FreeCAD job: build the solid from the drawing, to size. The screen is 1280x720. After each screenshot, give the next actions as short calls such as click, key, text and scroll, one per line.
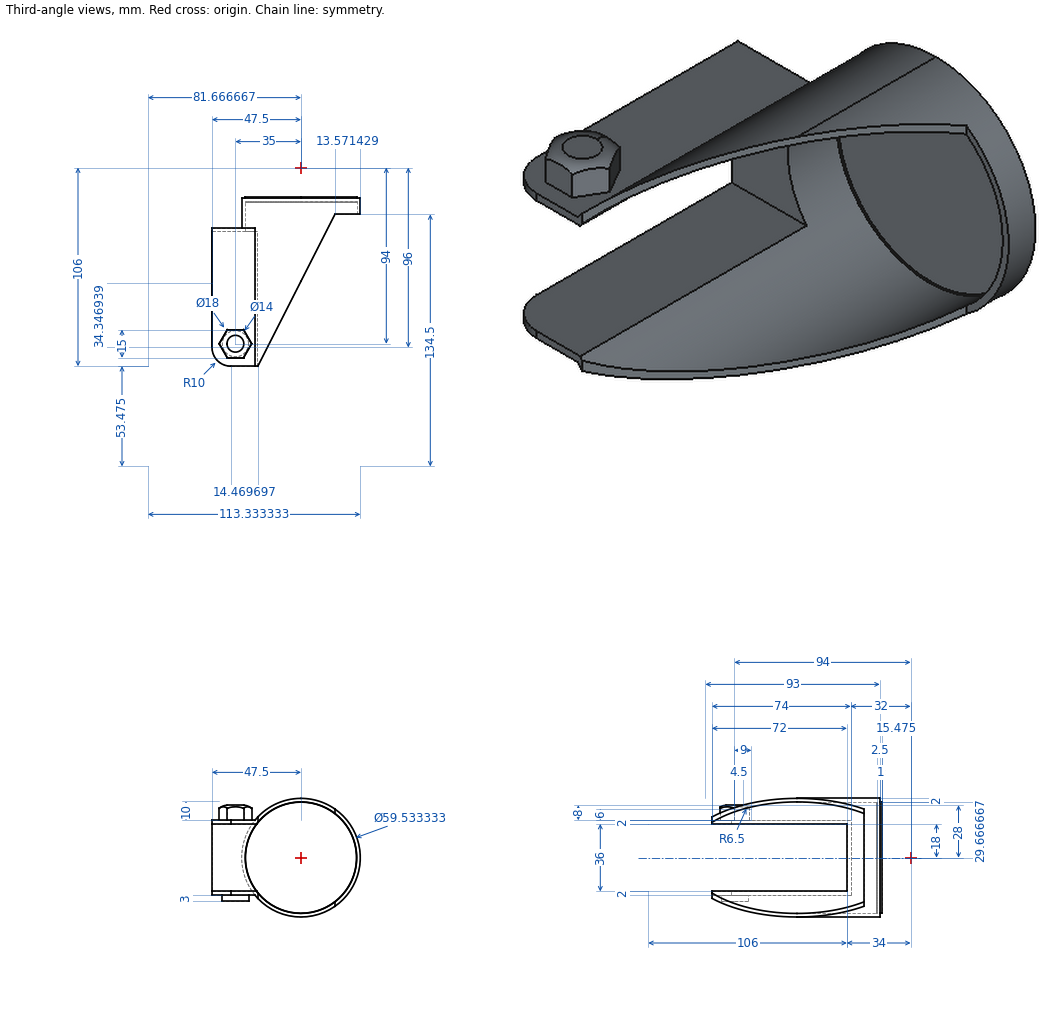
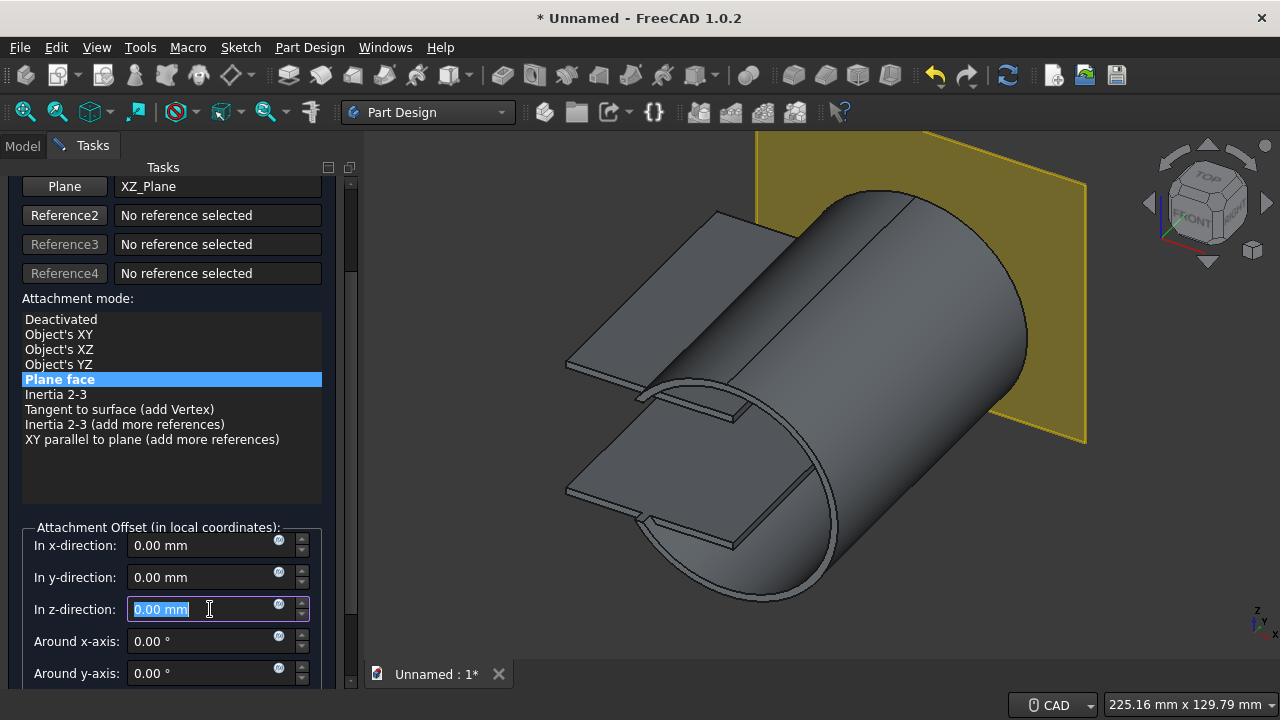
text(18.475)
key(Tab)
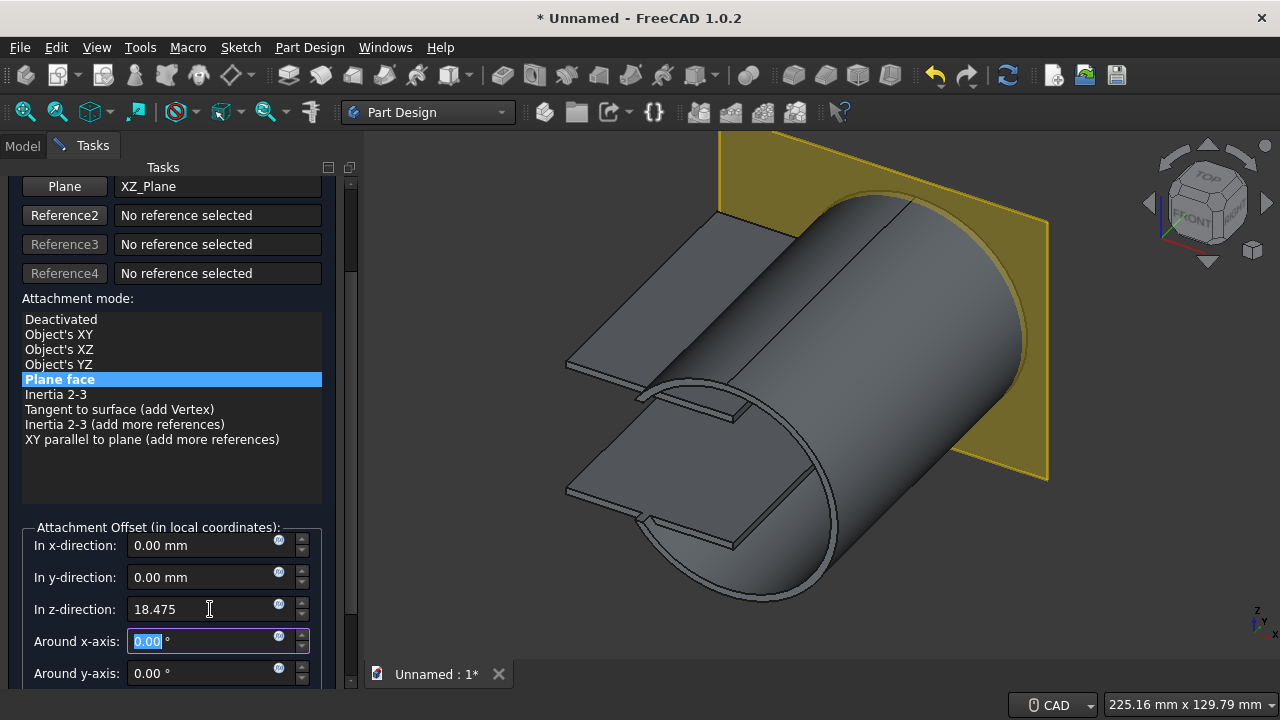
scroll(351, 432, up, 3)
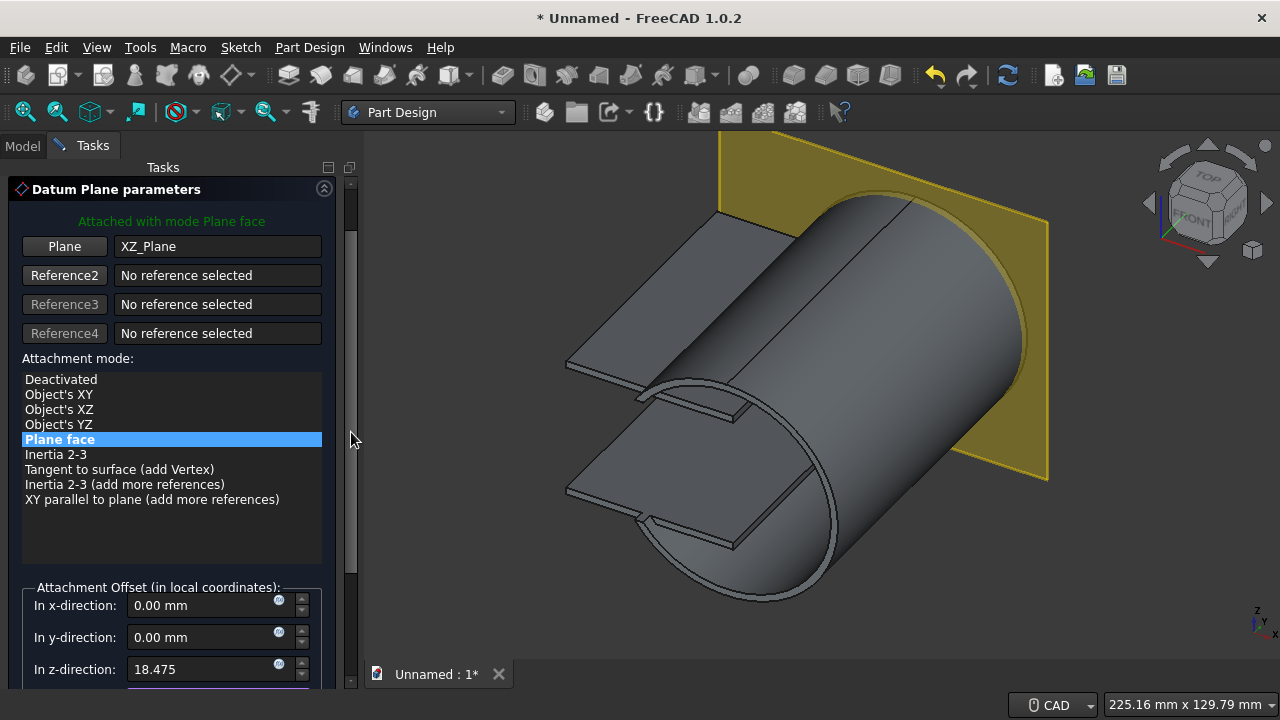
click(124, 206)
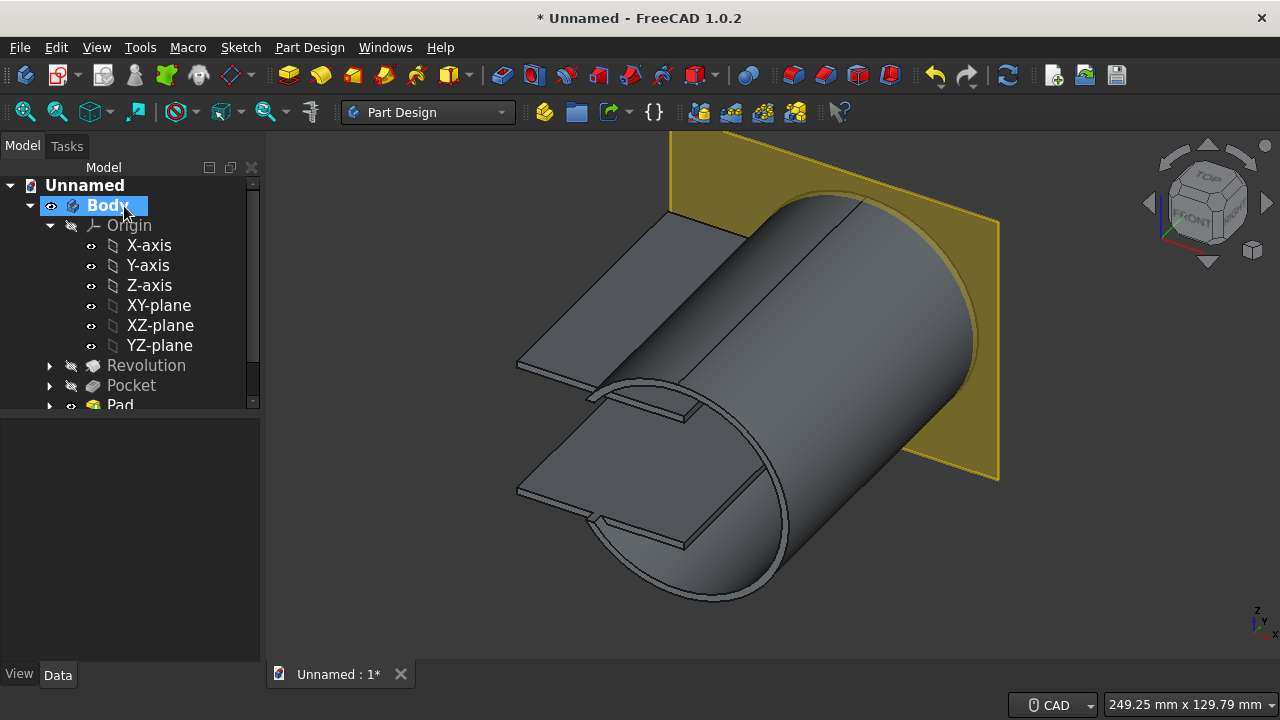
scroll(100, 301, down, 3)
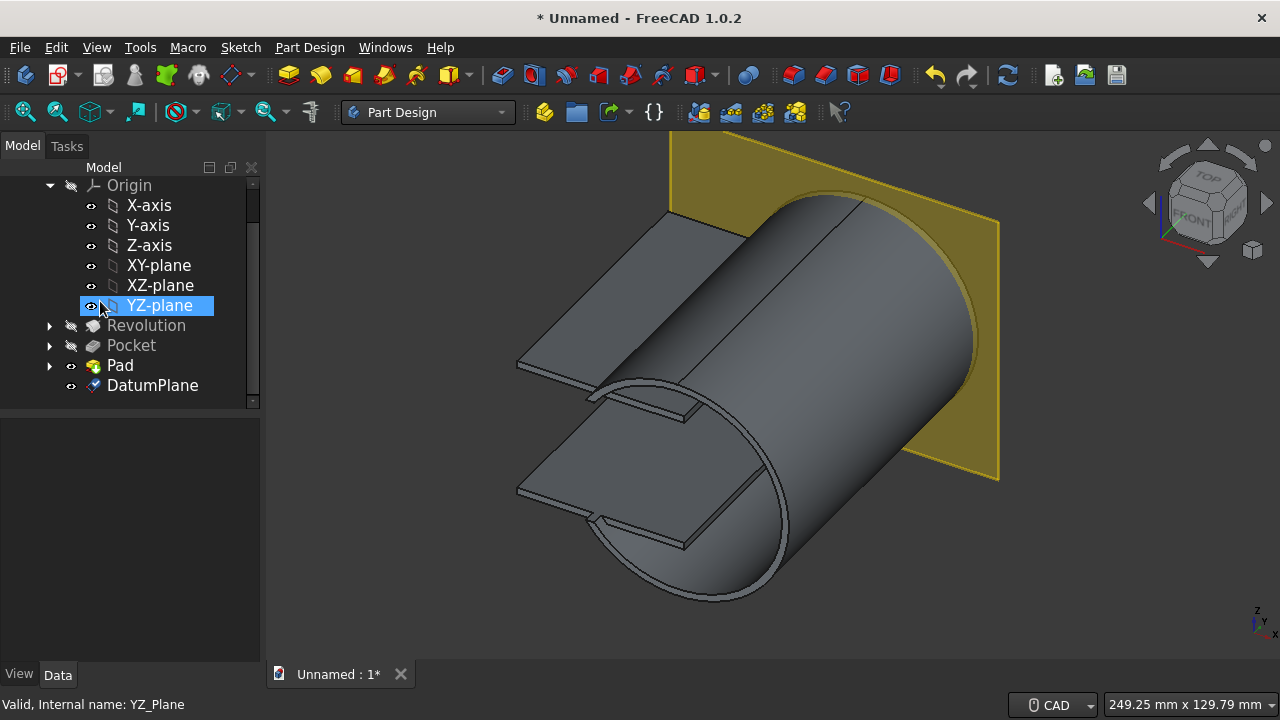
click(116, 386)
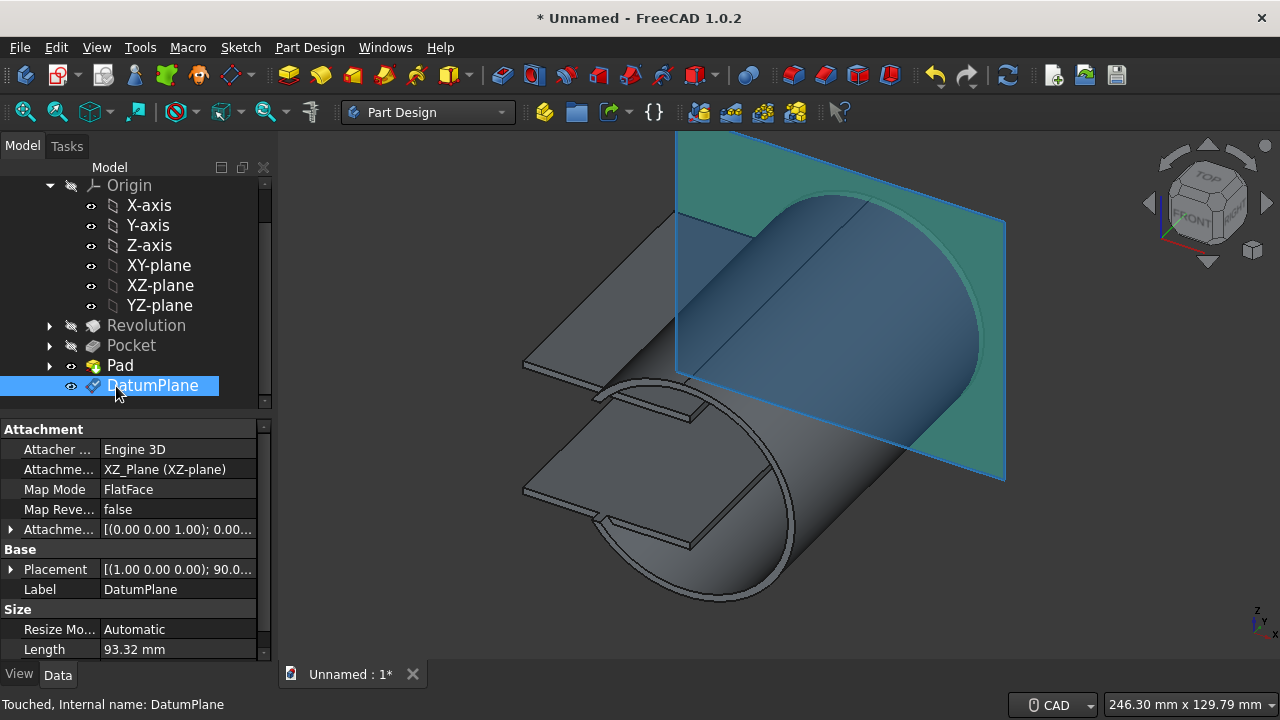
click(58, 76)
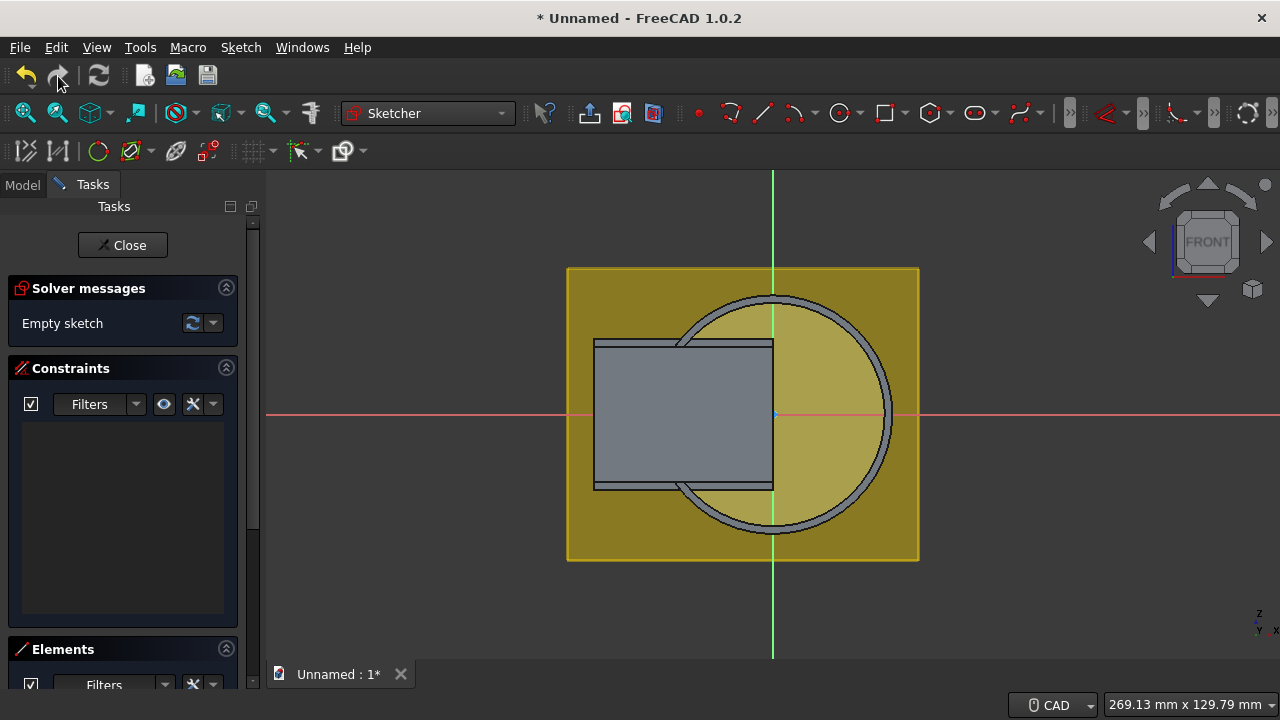
click(654, 114)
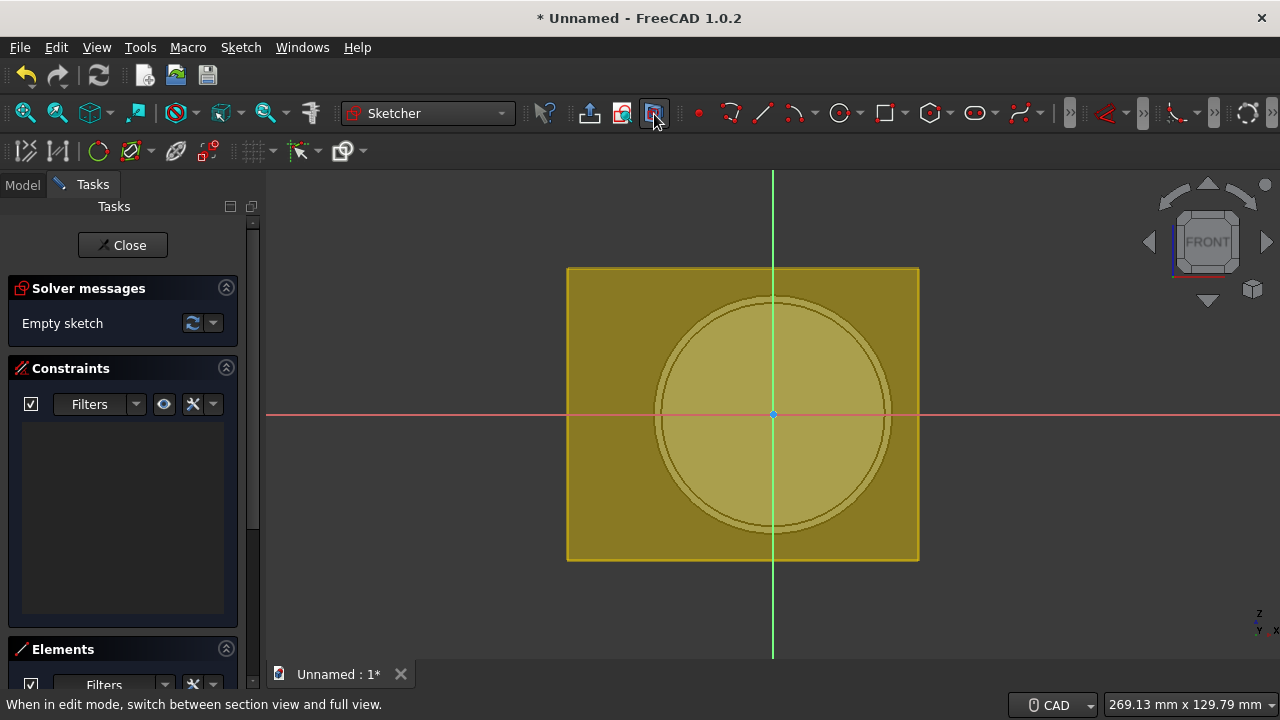
scroll(912, 415, up, 2)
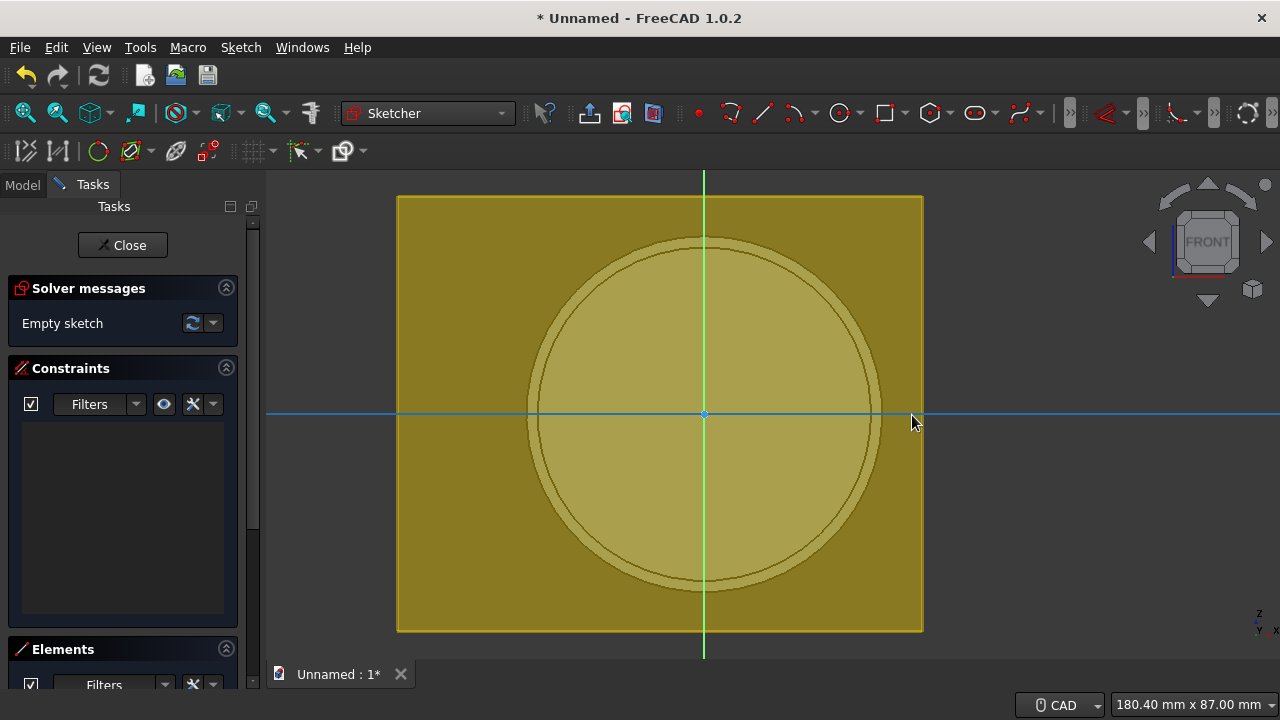
key(g)
key(c)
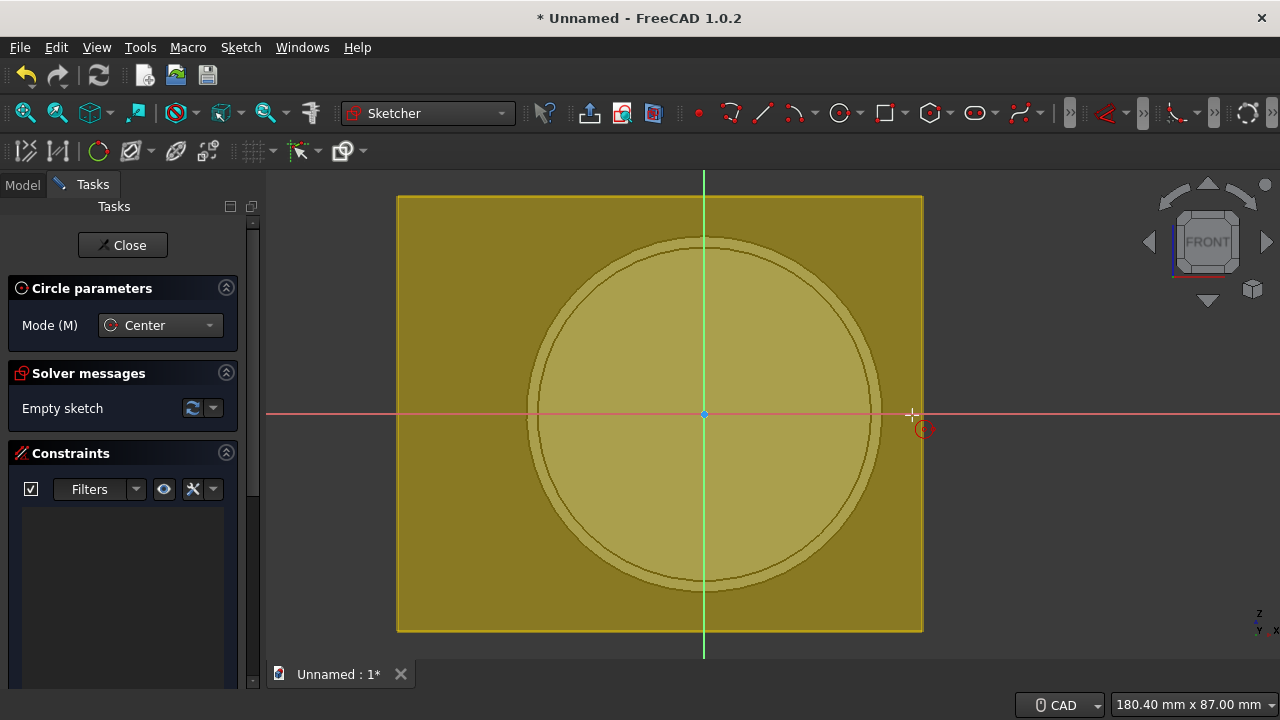
click(704, 414)
click(823, 296)
key(Escape)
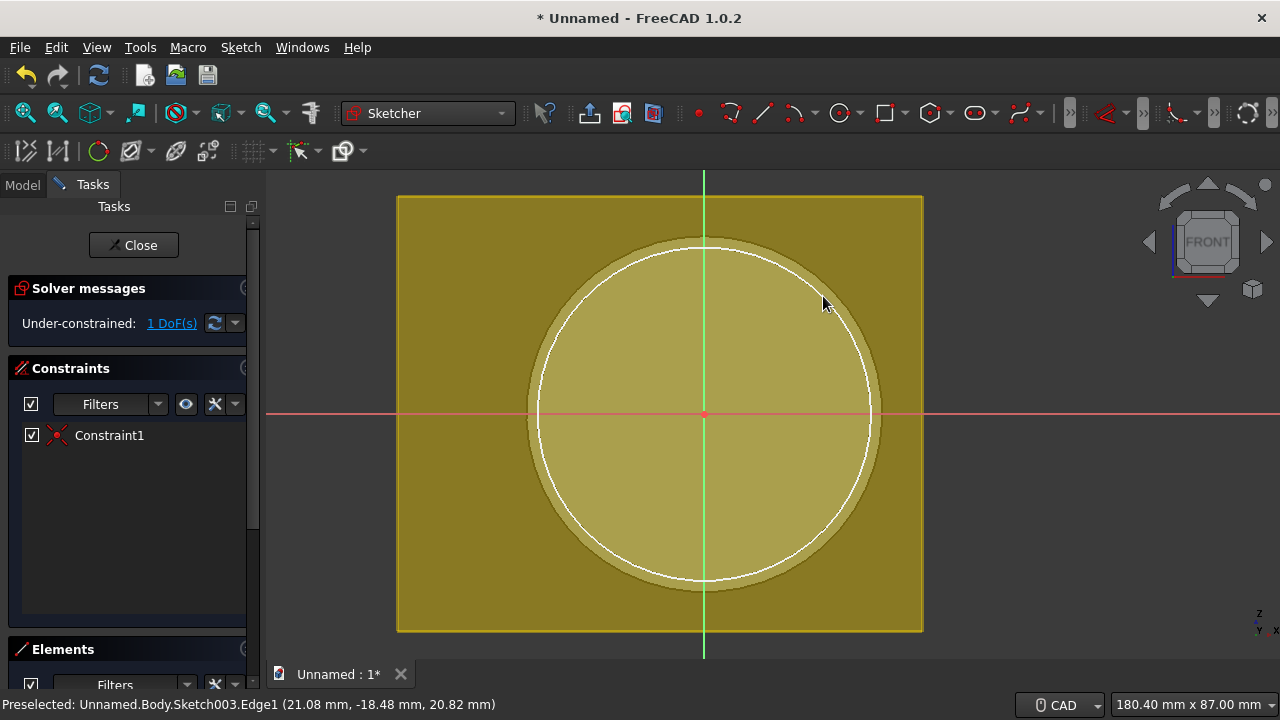
key(d)